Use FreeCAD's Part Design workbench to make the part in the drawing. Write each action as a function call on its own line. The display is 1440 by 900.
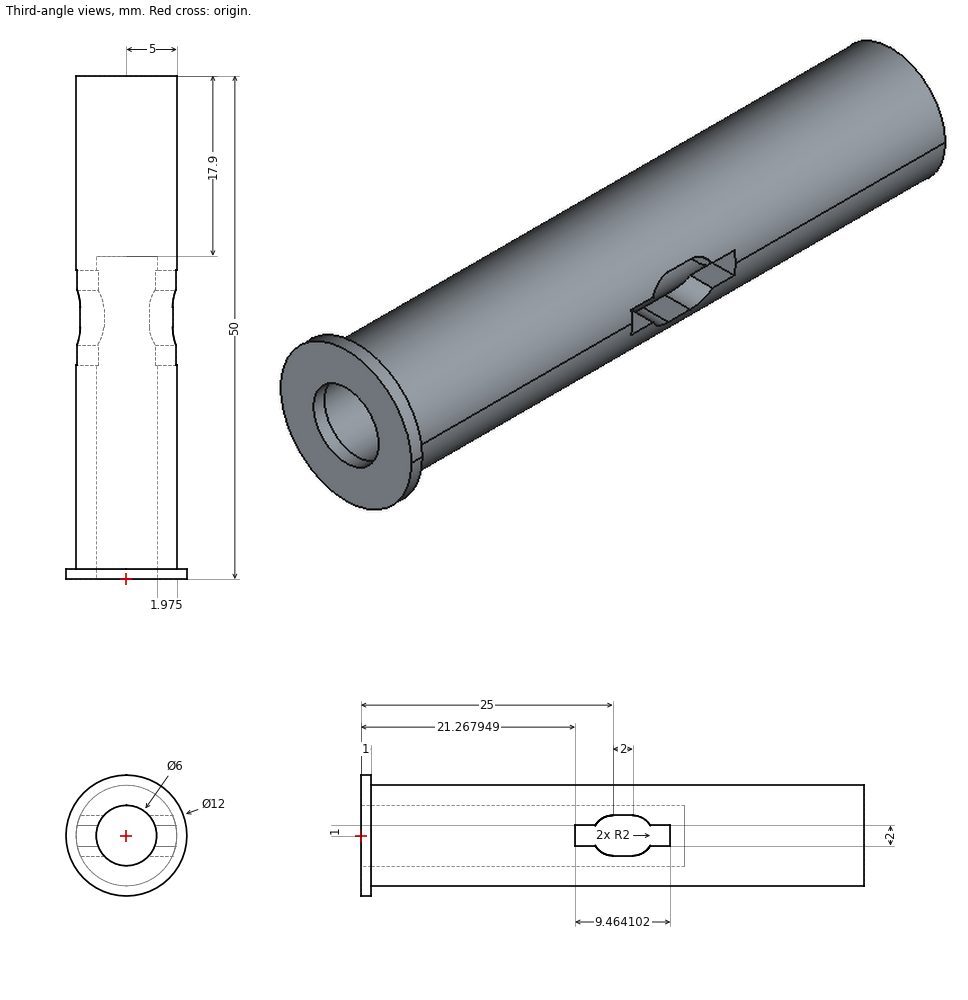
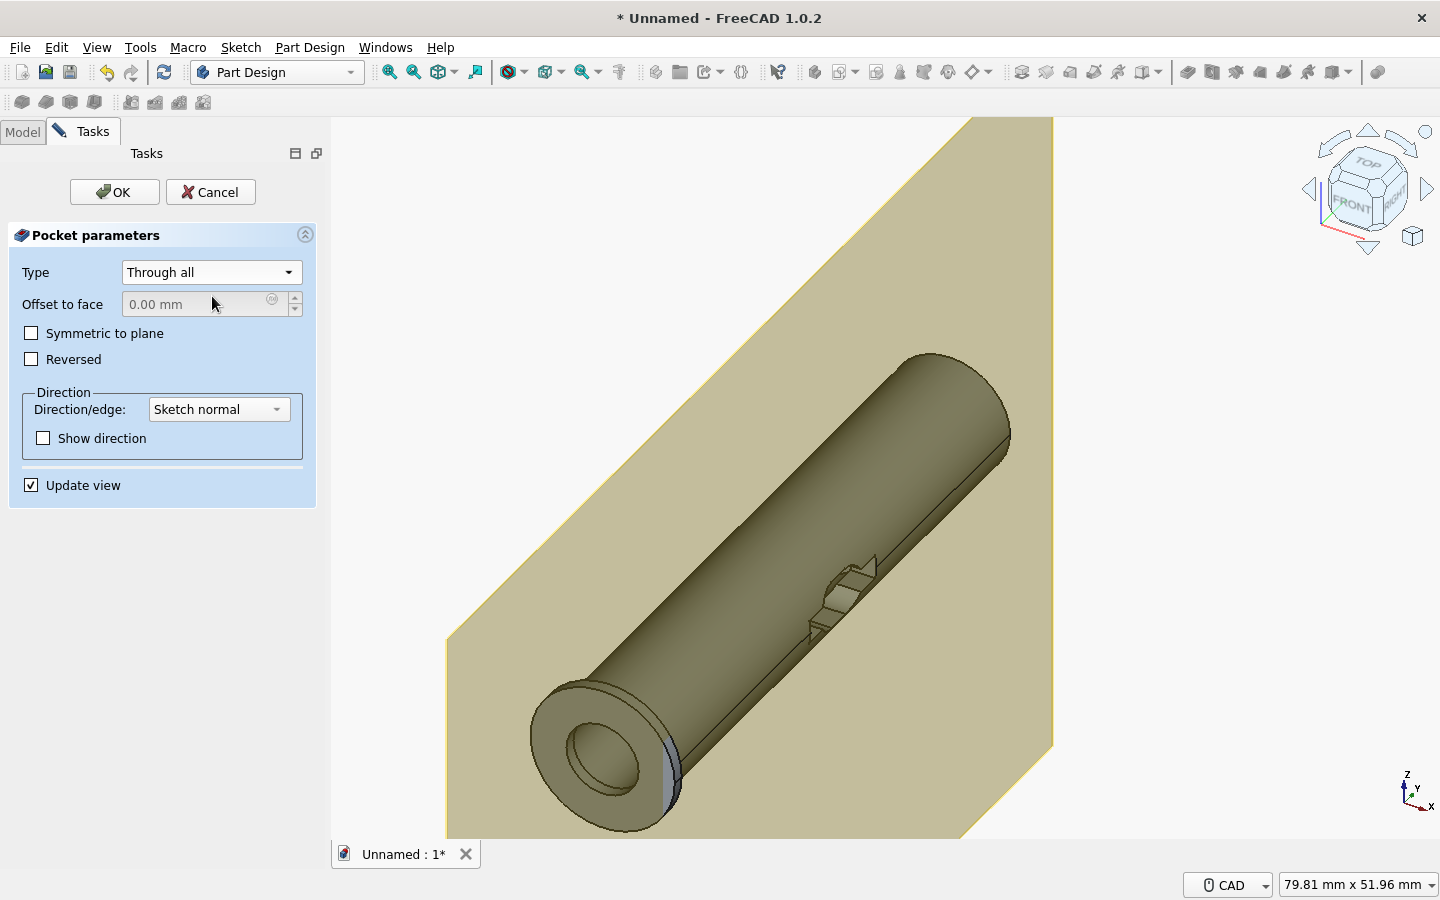
click(115, 192)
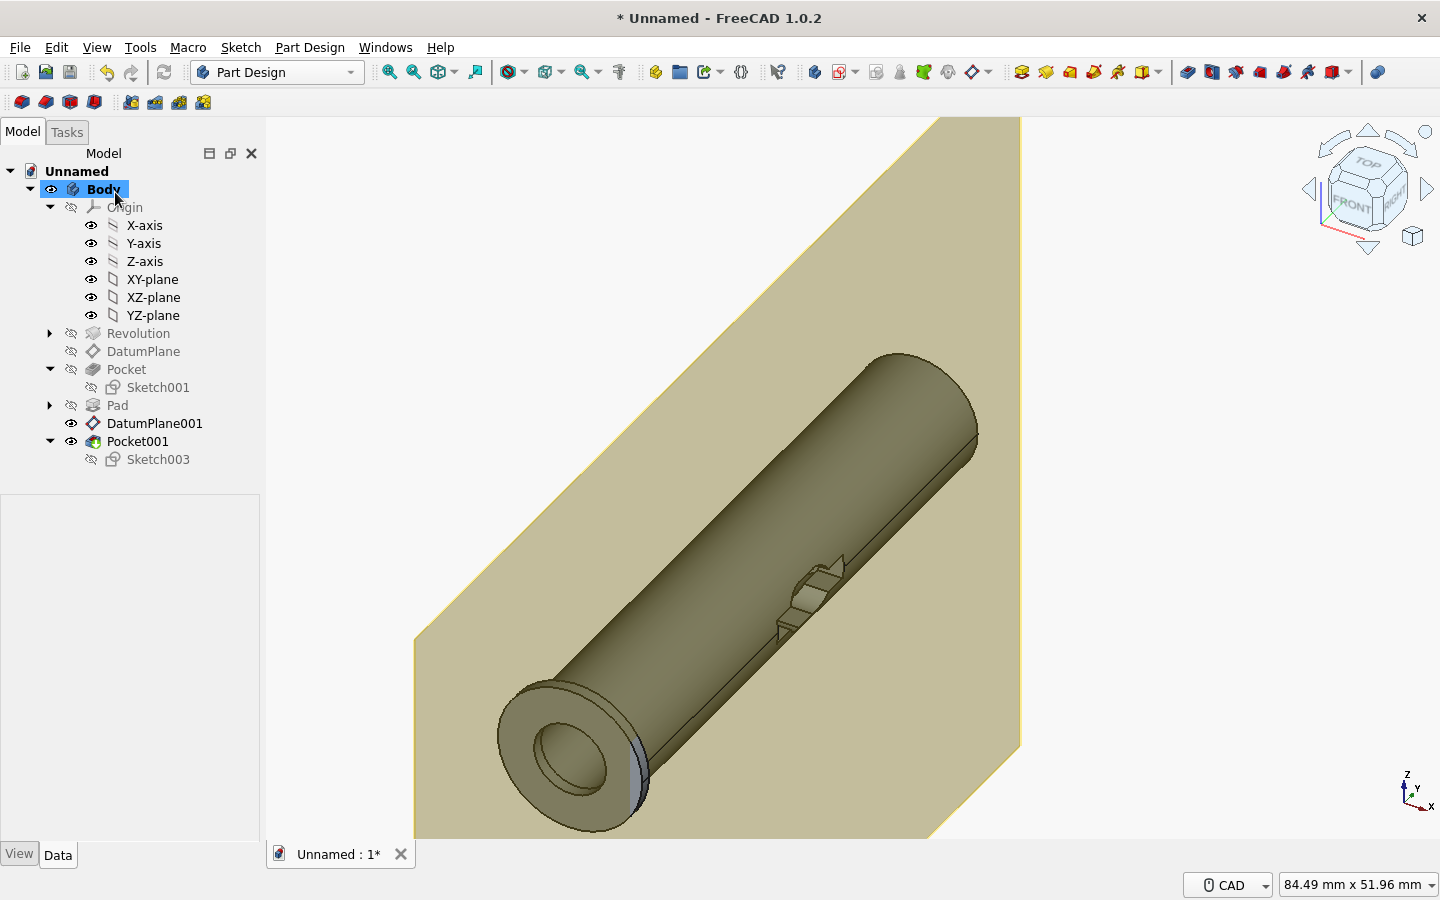
click(116, 423)
key(space)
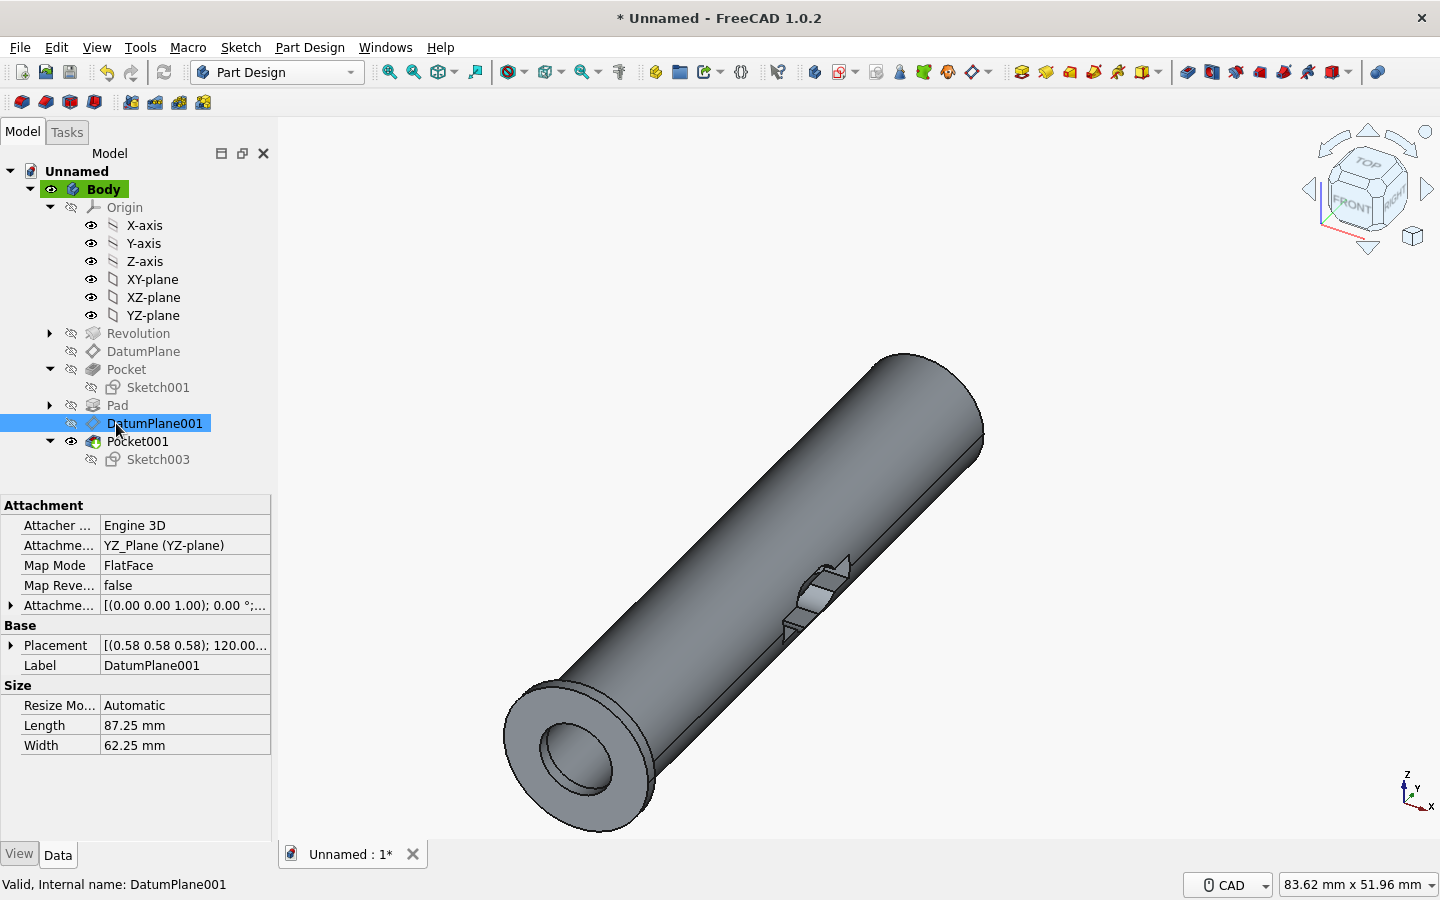
key(0)